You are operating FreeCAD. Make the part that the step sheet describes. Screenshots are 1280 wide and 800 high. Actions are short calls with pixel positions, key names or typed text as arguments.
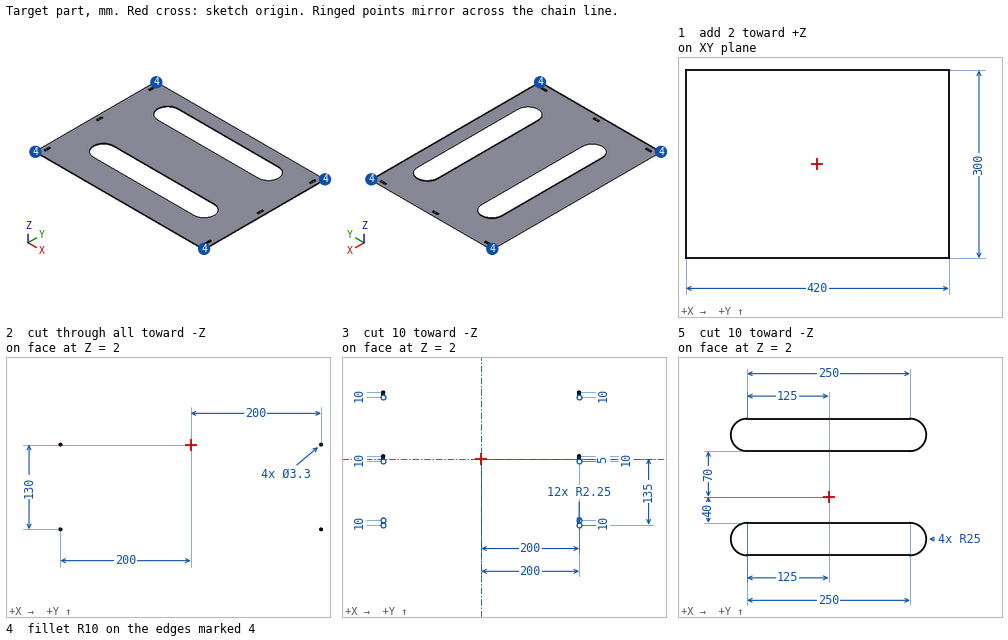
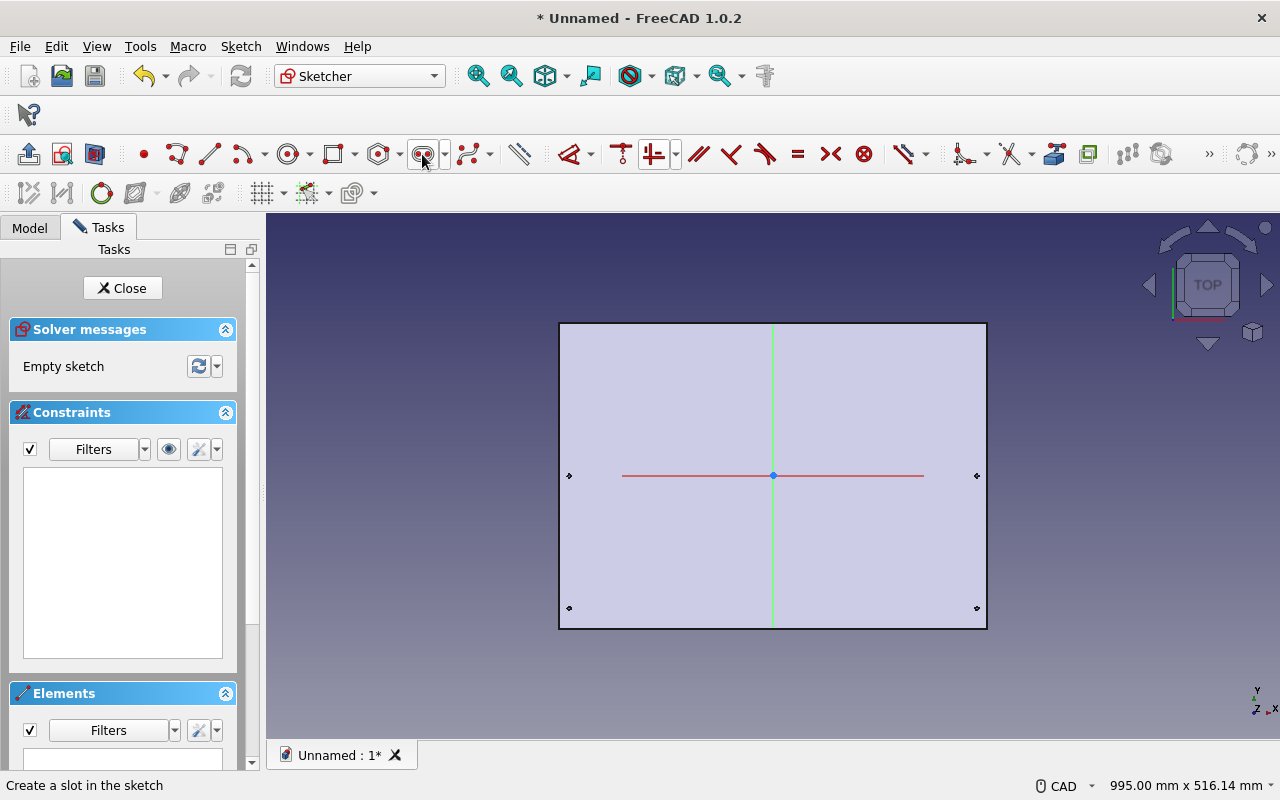
scroll(977, 614, up, 12)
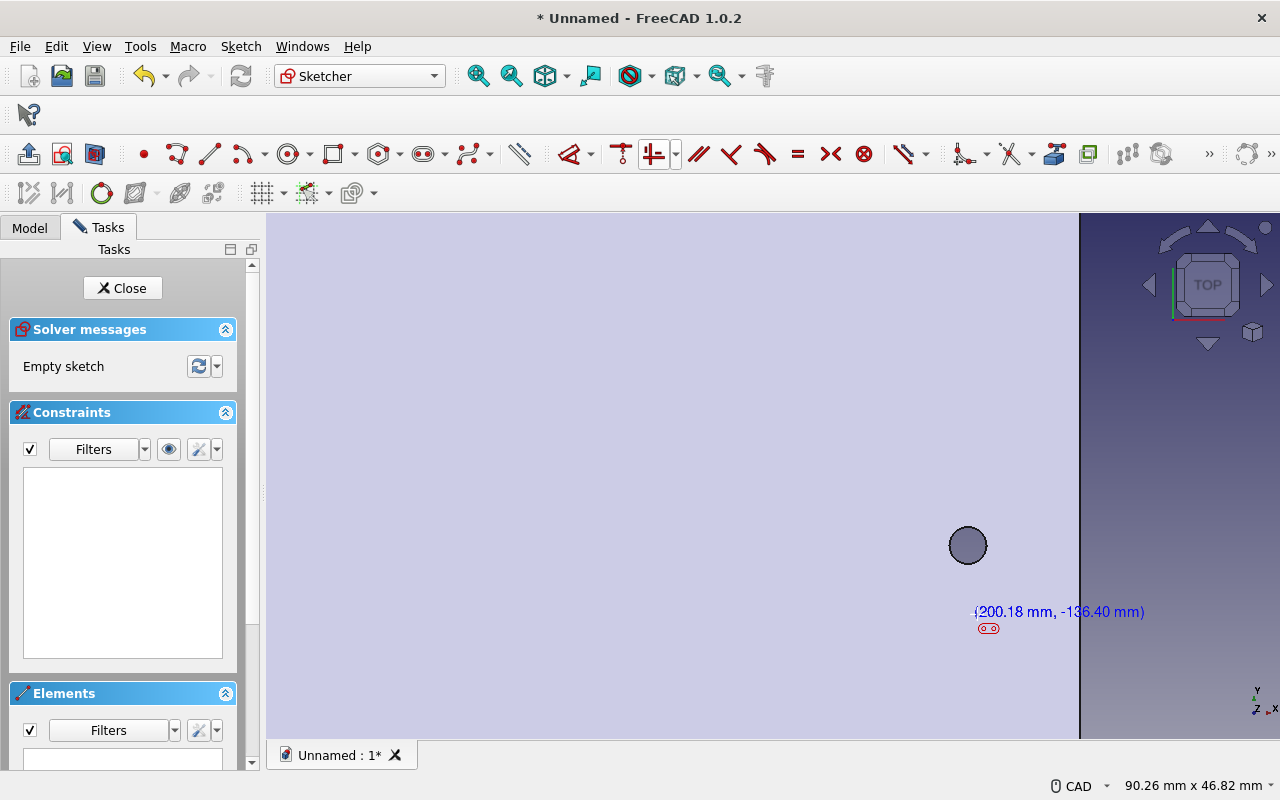
scroll(952, 649, down, 11)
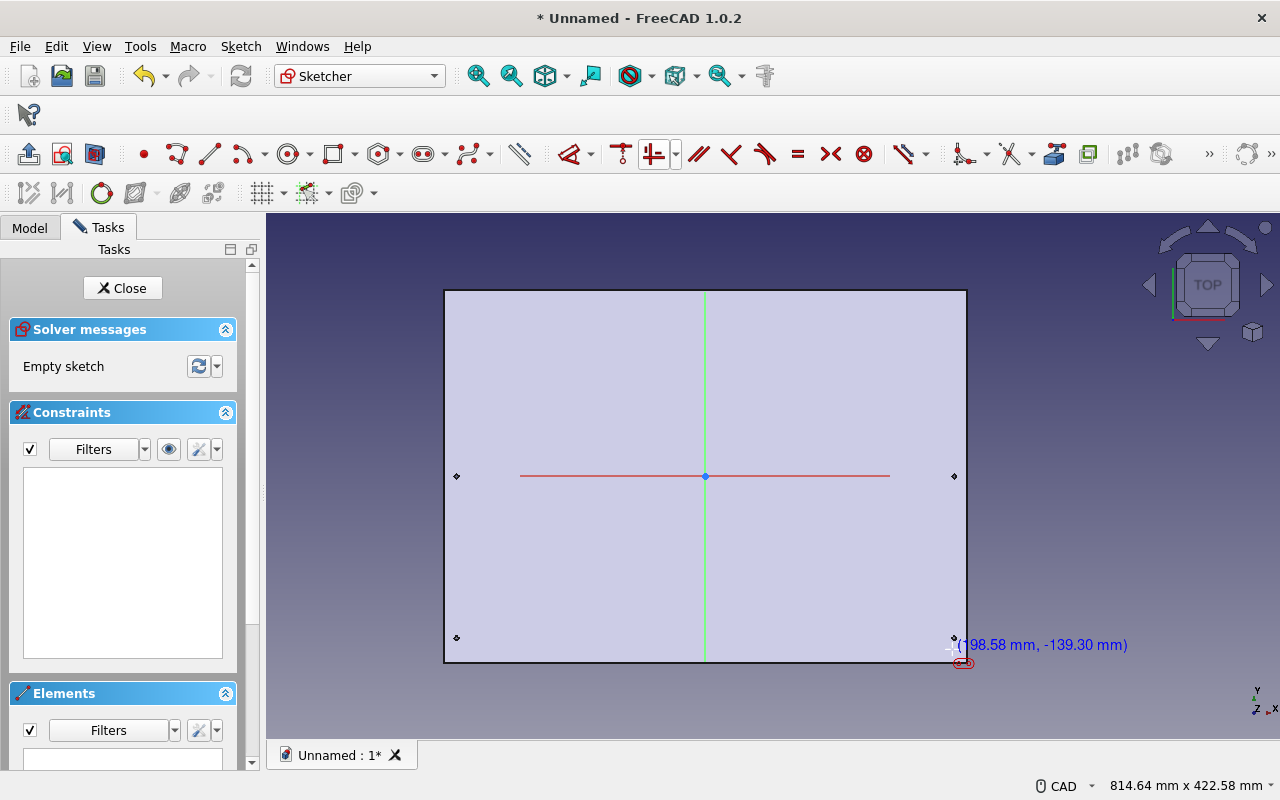
click(954, 644)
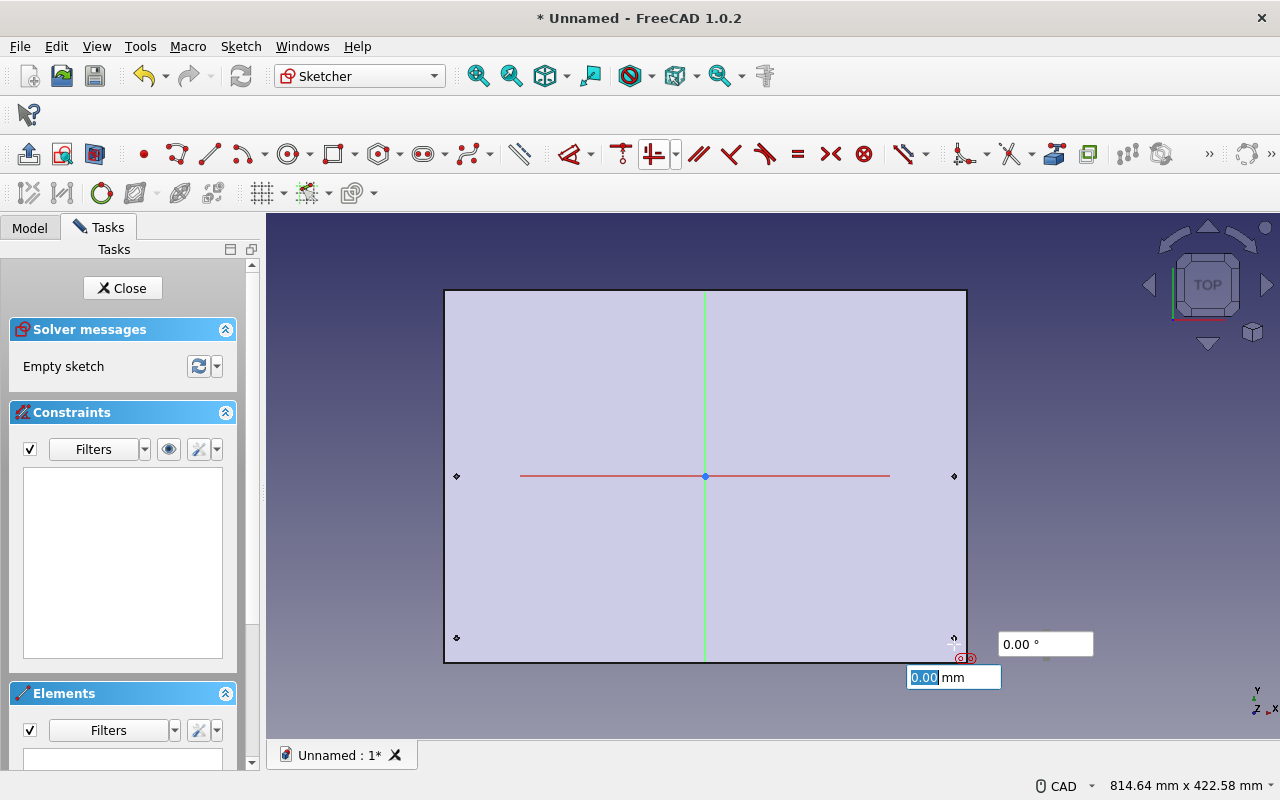
scroll(954, 632, up, 2)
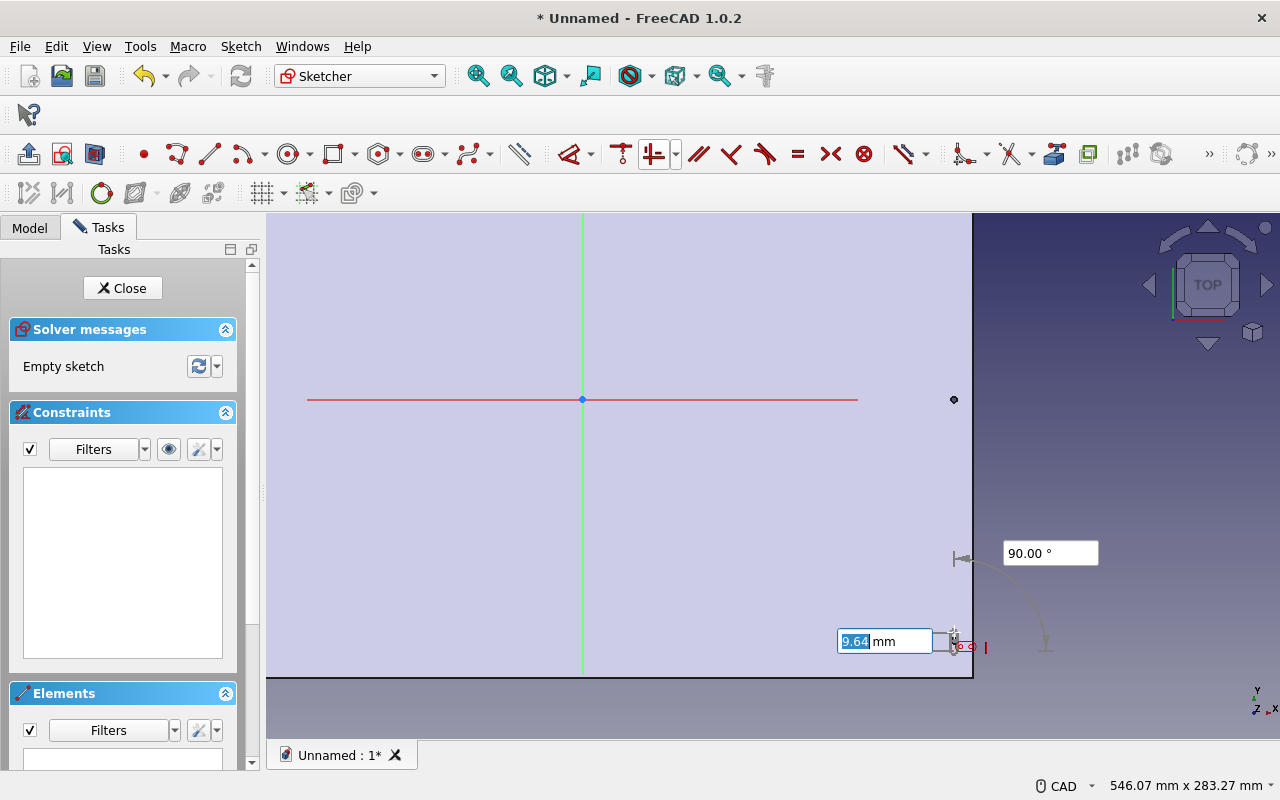
click(954, 632)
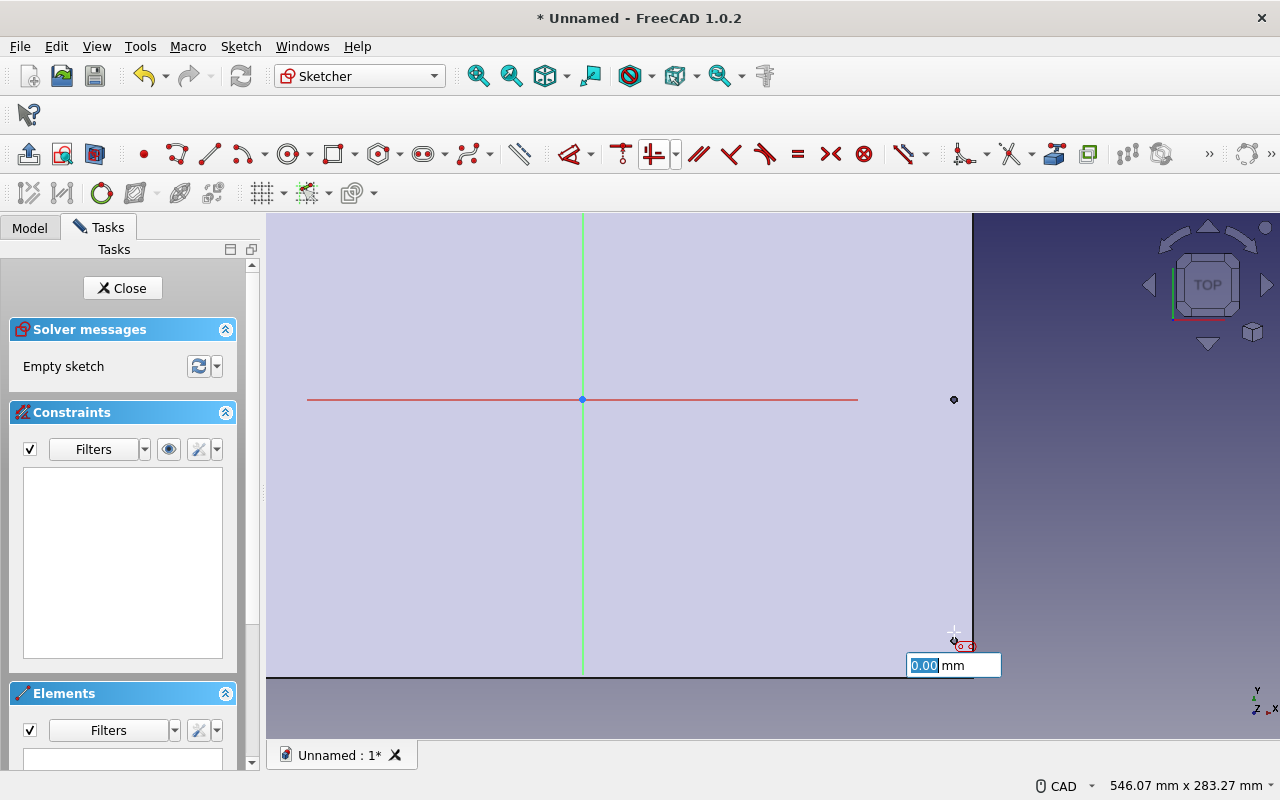
scroll(950, 641, up, 7)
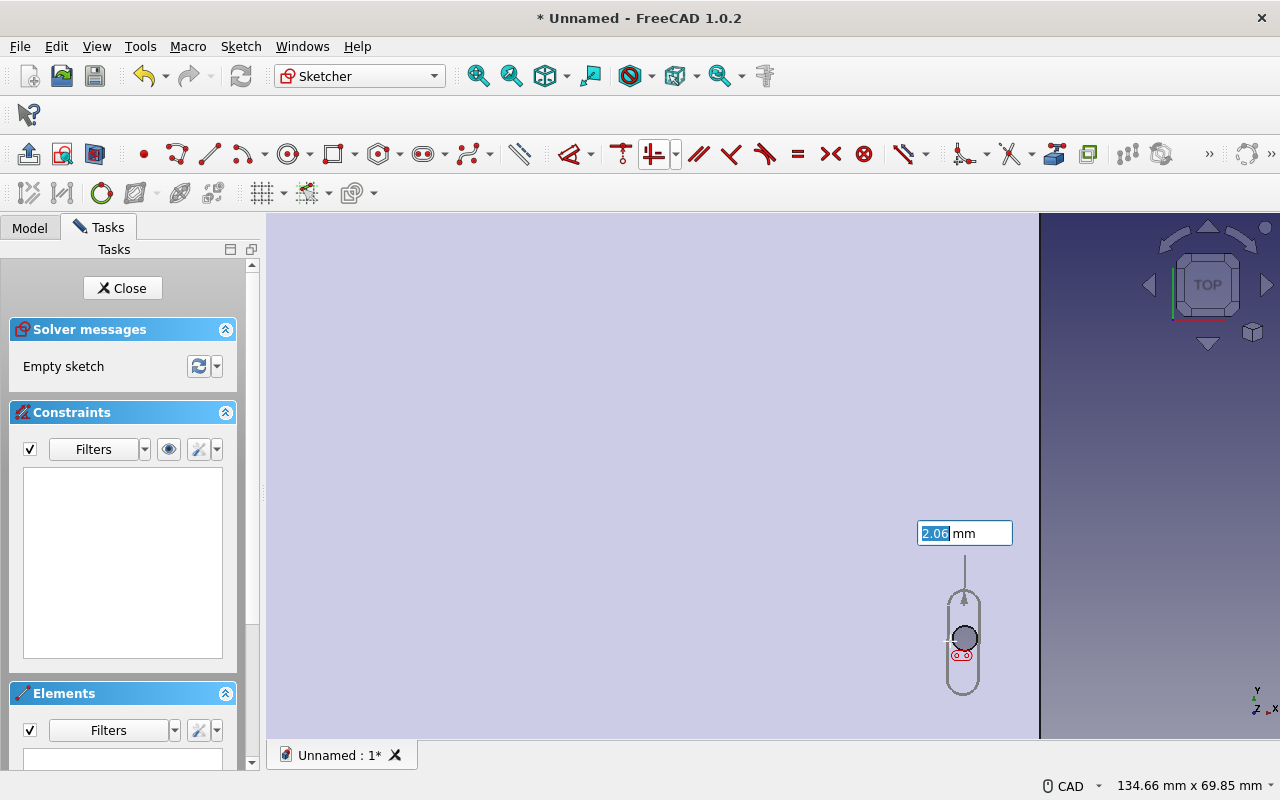
click(948, 638)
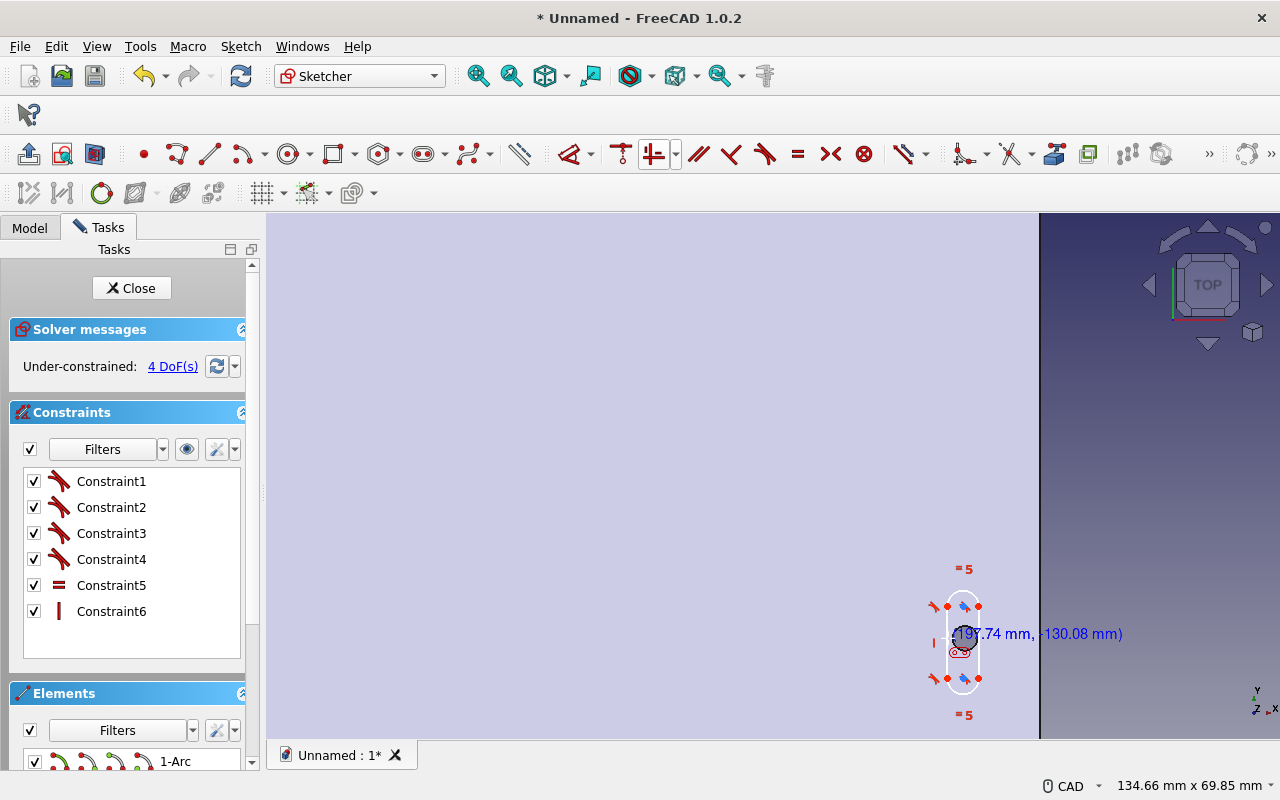
scroll(951, 638, down, 9)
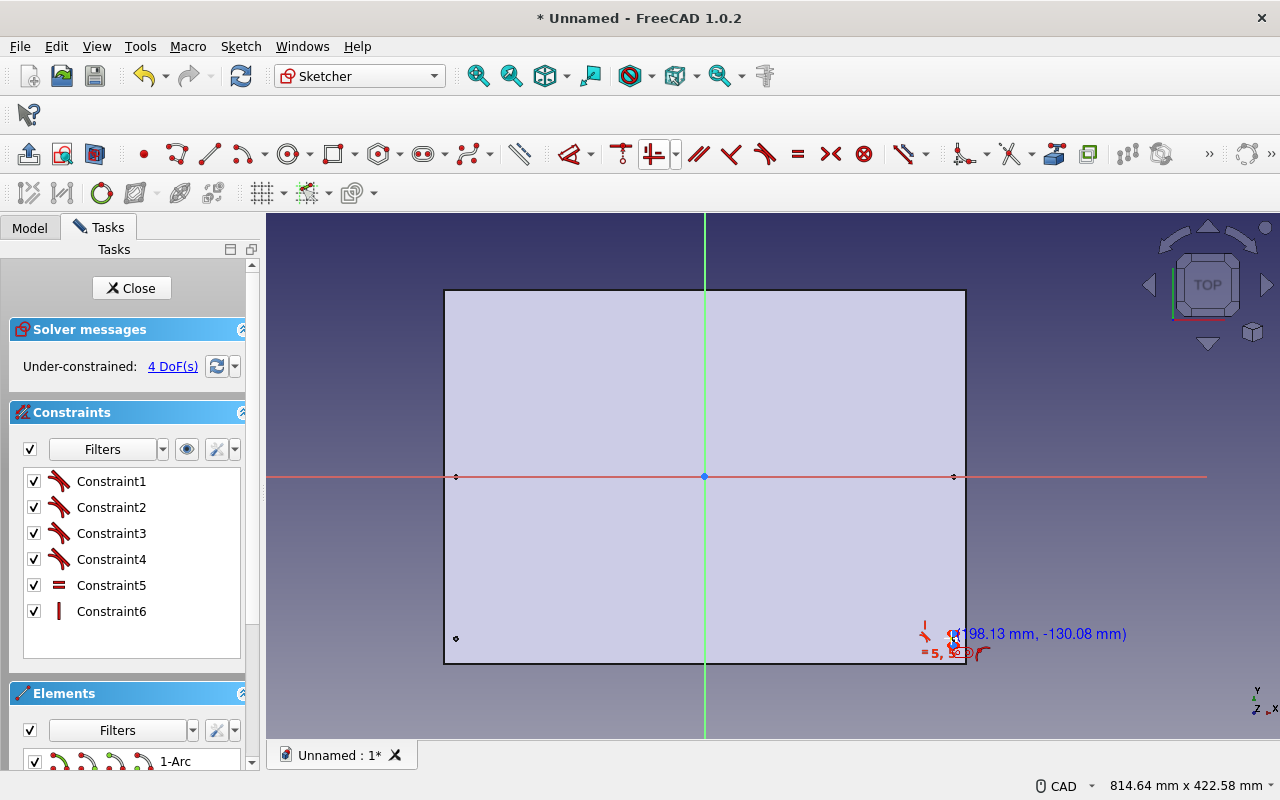
scroll(456, 645, up, 11)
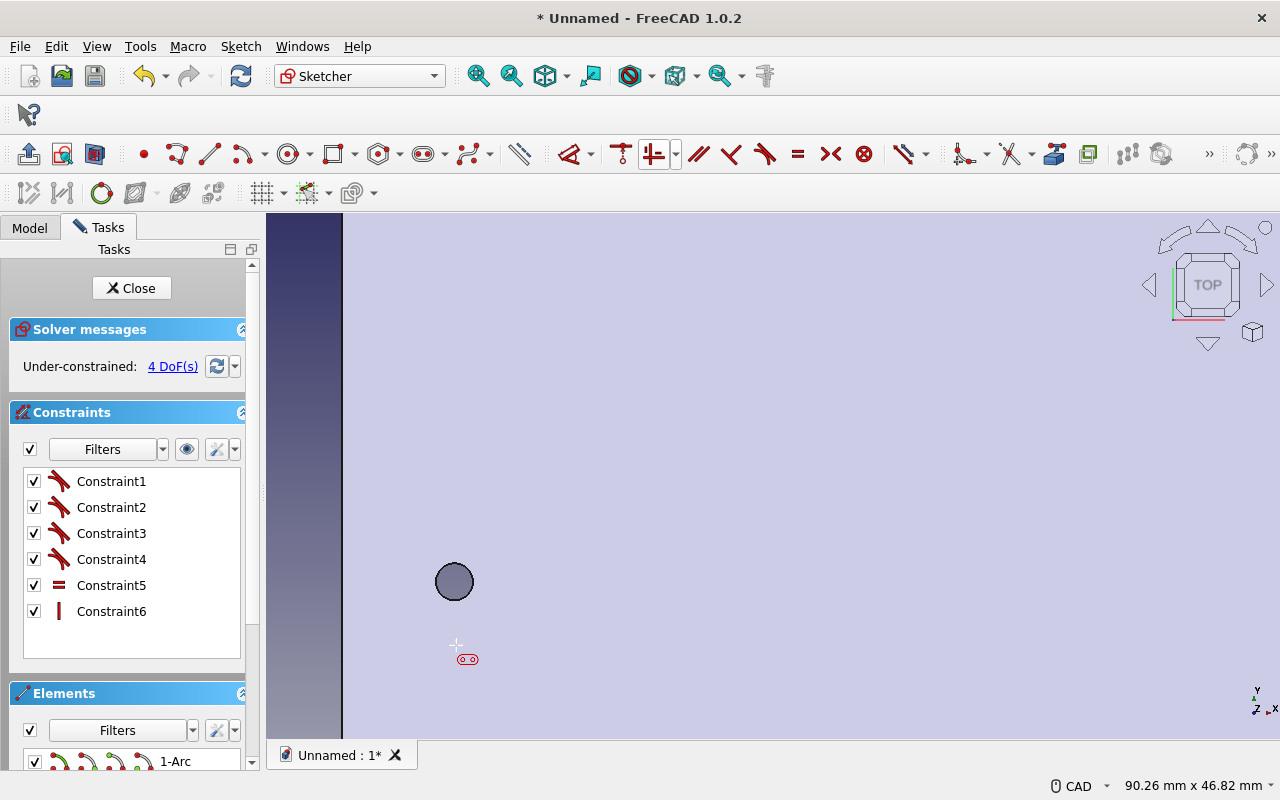
scroll(456, 645, down, 11)